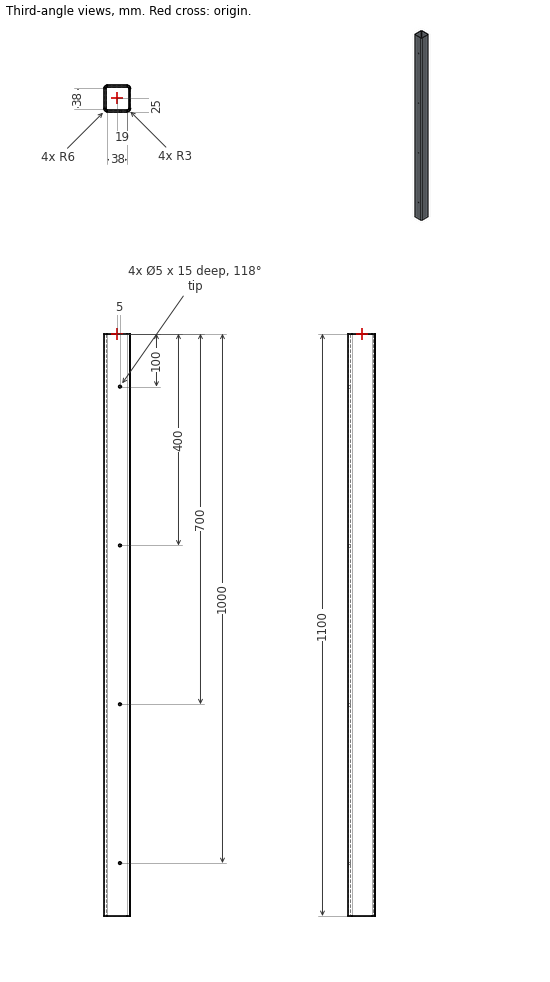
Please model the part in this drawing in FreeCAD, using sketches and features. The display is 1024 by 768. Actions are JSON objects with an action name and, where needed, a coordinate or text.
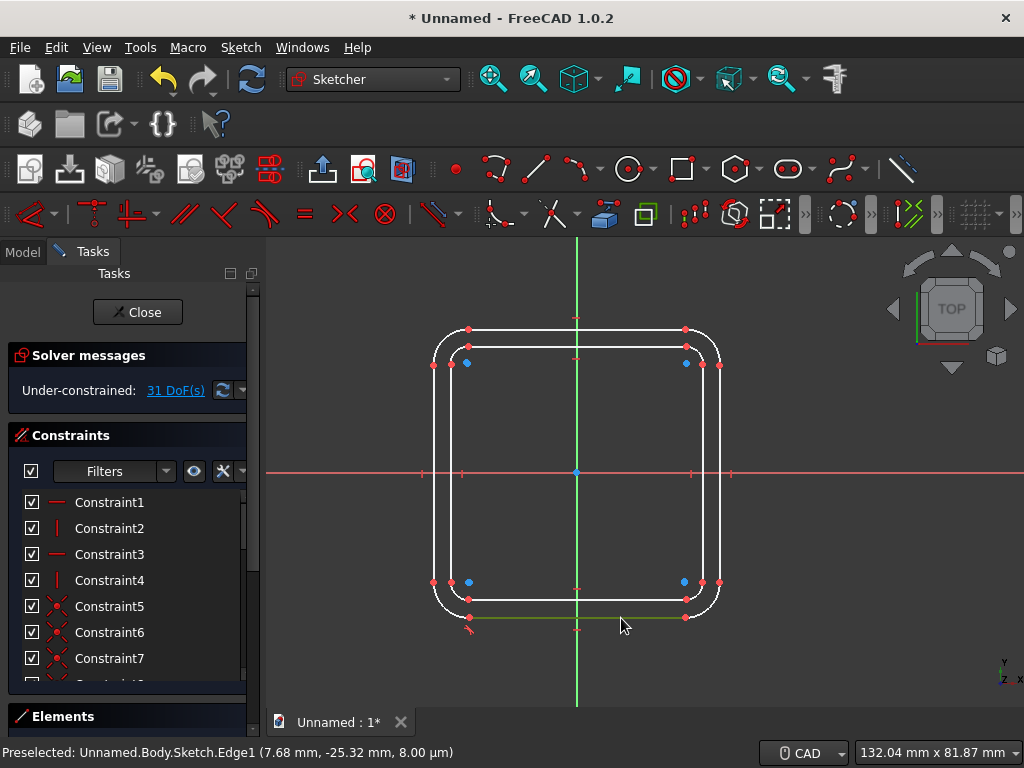
{"action": "left_click", "coordinate": [701, 614]}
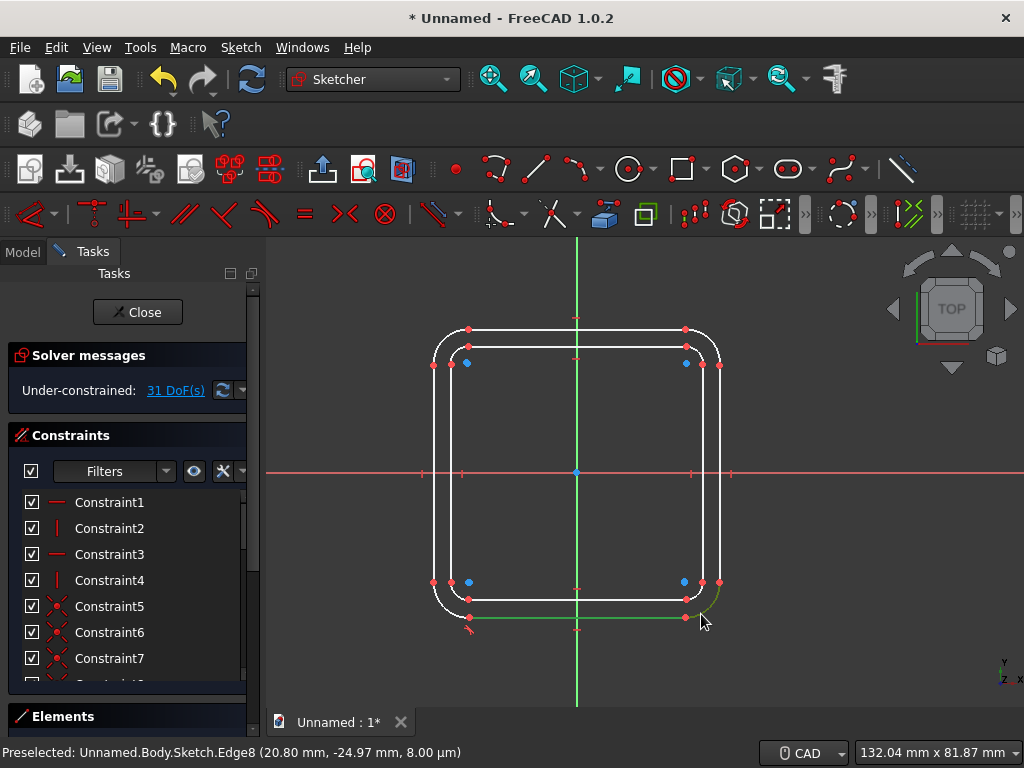
{"action": "left_click", "coordinate": [266, 214]}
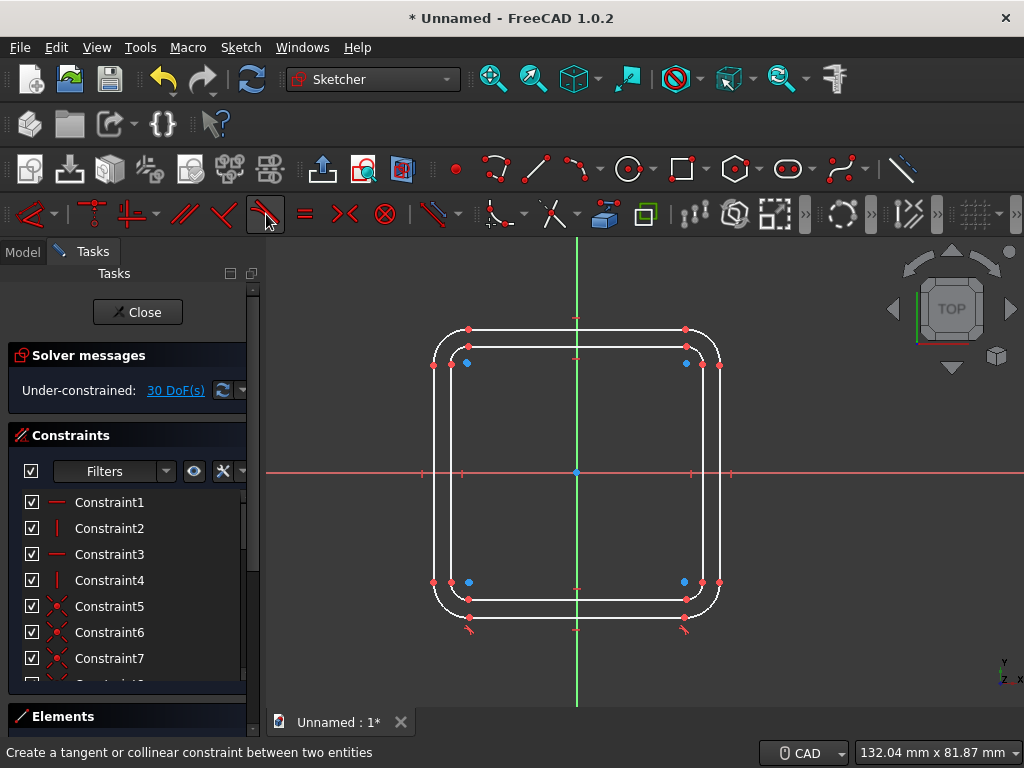
{"action": "left_click", "coordinate": [434, 517]}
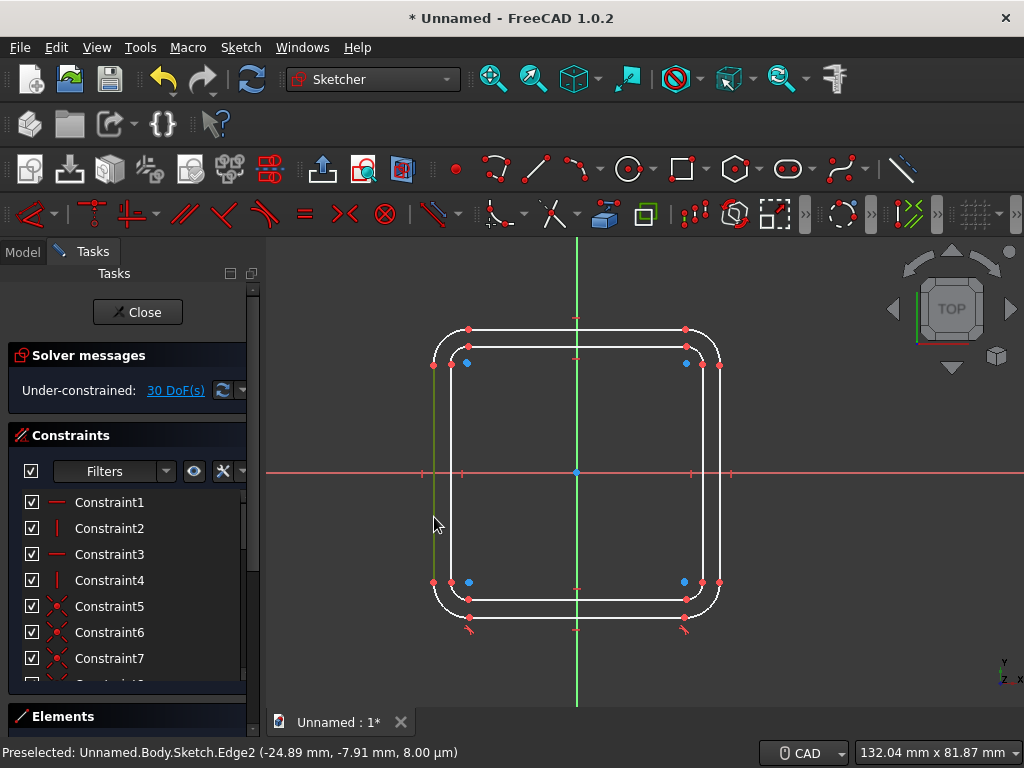
{"action": "left_click", "coordinate": [438, 599]}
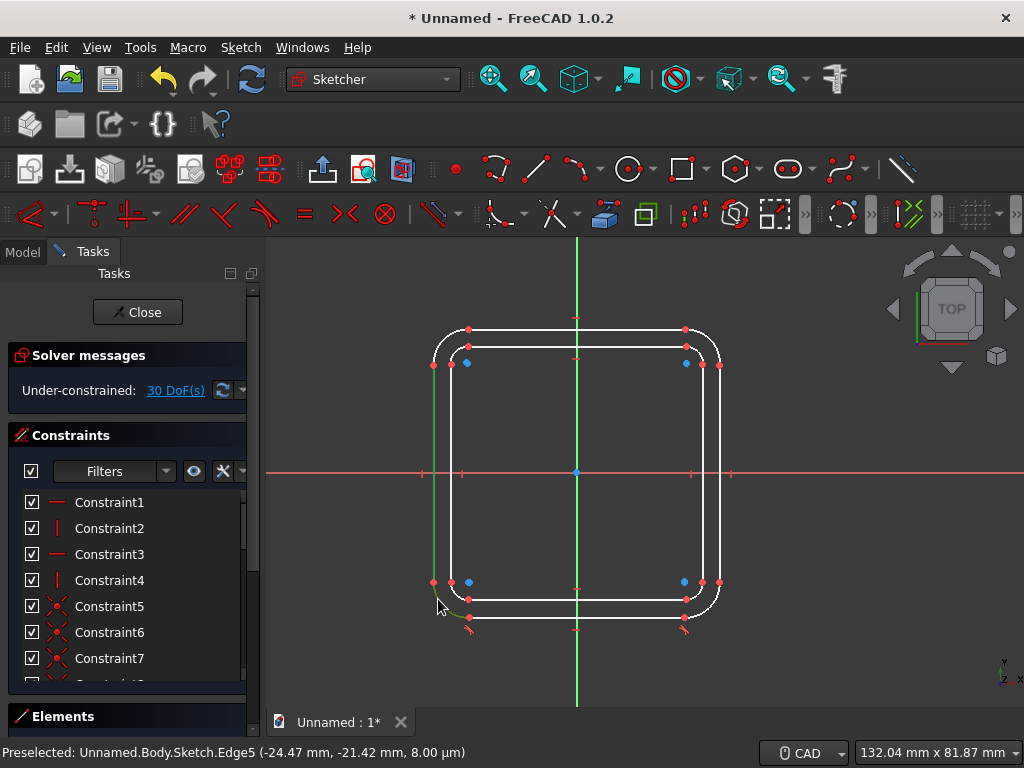
{"action": "left_click", "coordinate": [266, 214]}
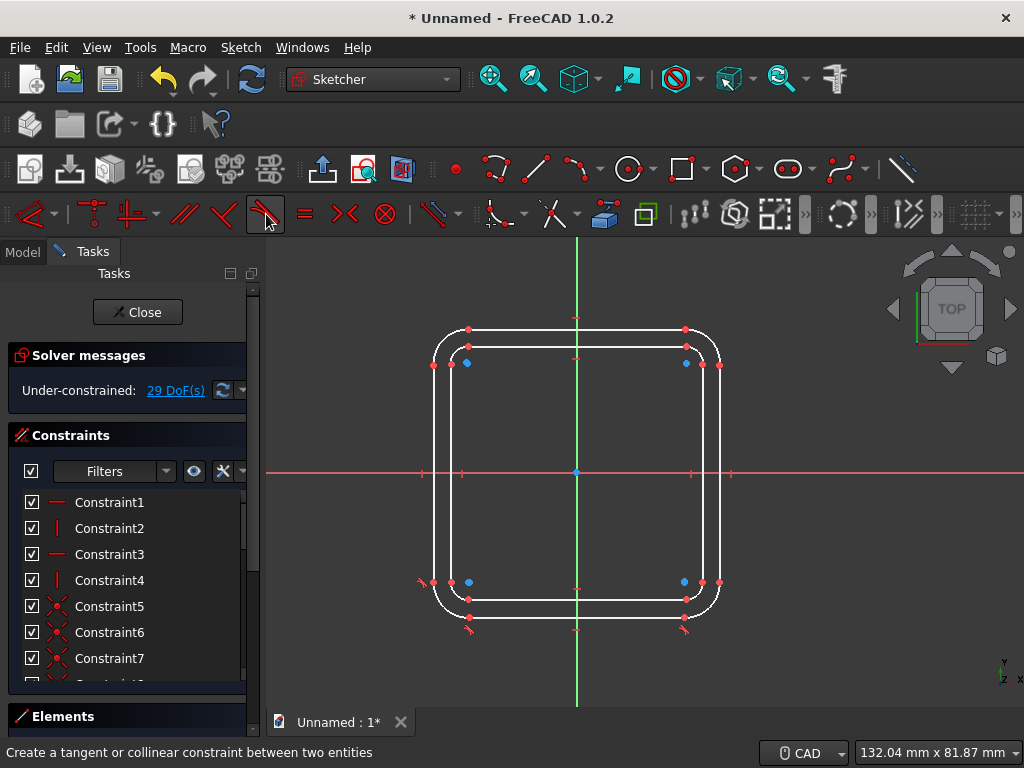
{"action": "left_click", "coordinate": [434, 517]}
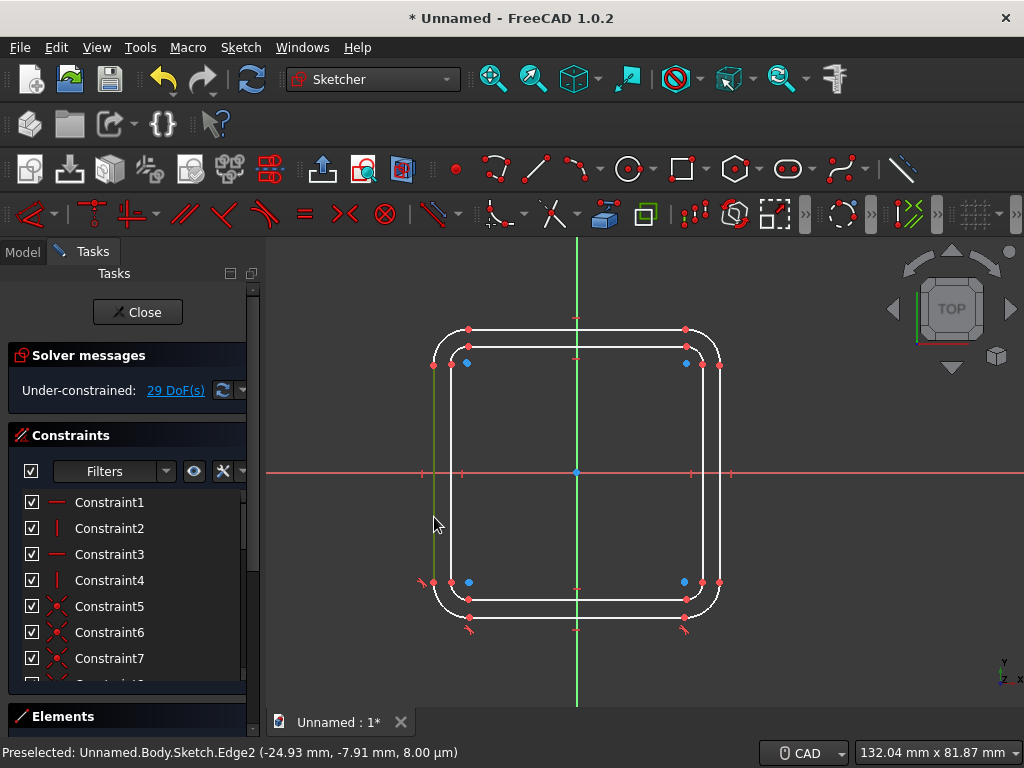
{"action": "left_click", "coordinate": [452, 333]}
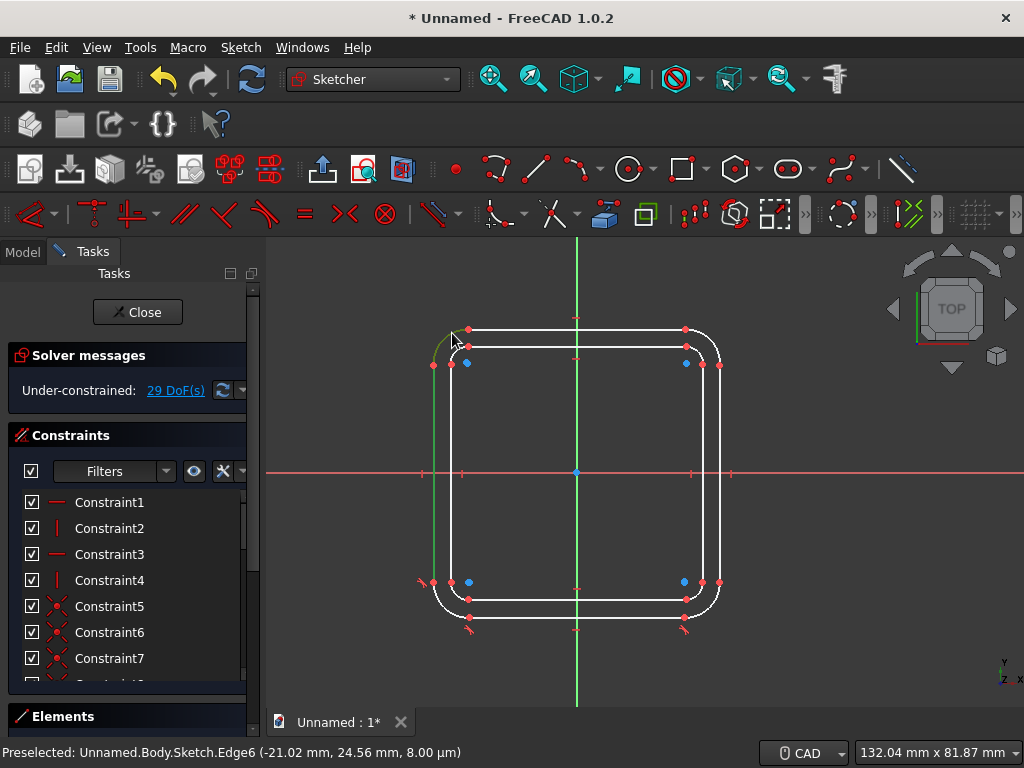
{"action": "key", "text": "t"}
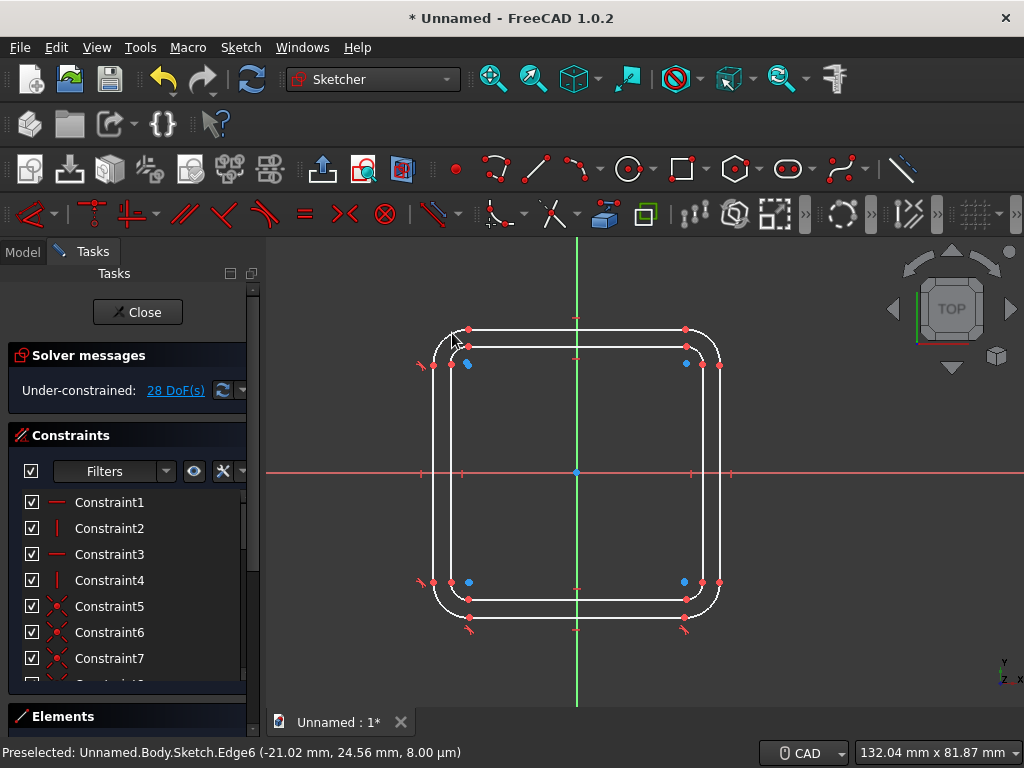
{"action": "left_click", "coordinate": [533, 330]}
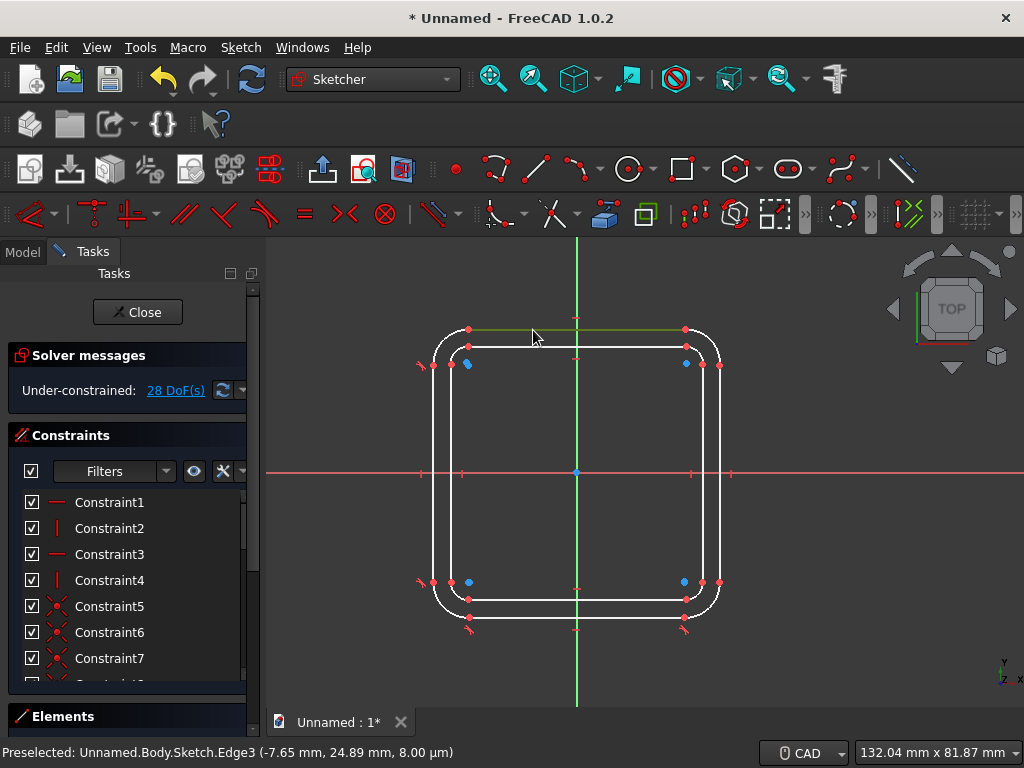
{"action": "left_click", "coordinate": [452, 334]}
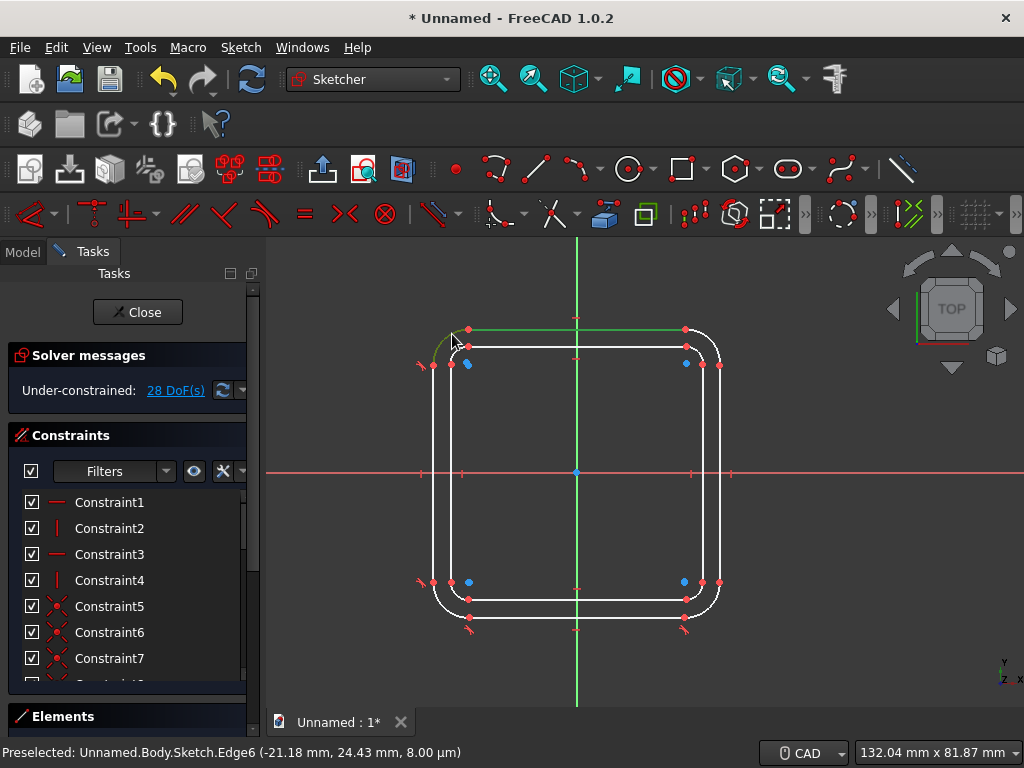
{"action": "key", "text": "t"}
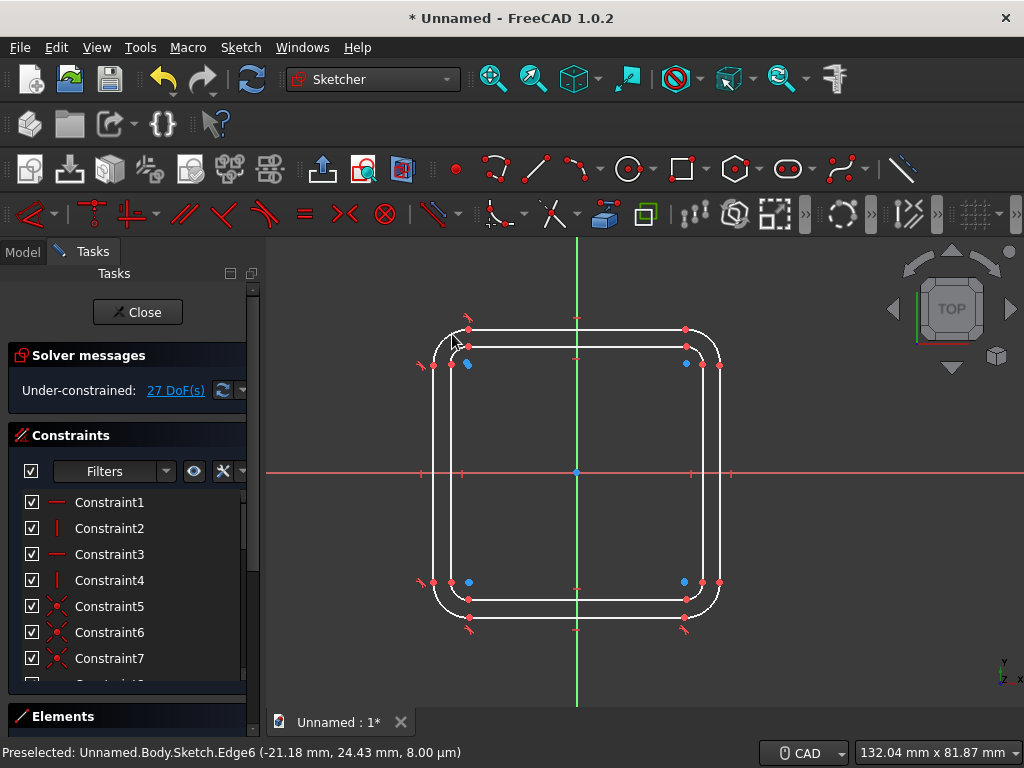
{"action": "left_click", "coordinate": [534, 330]}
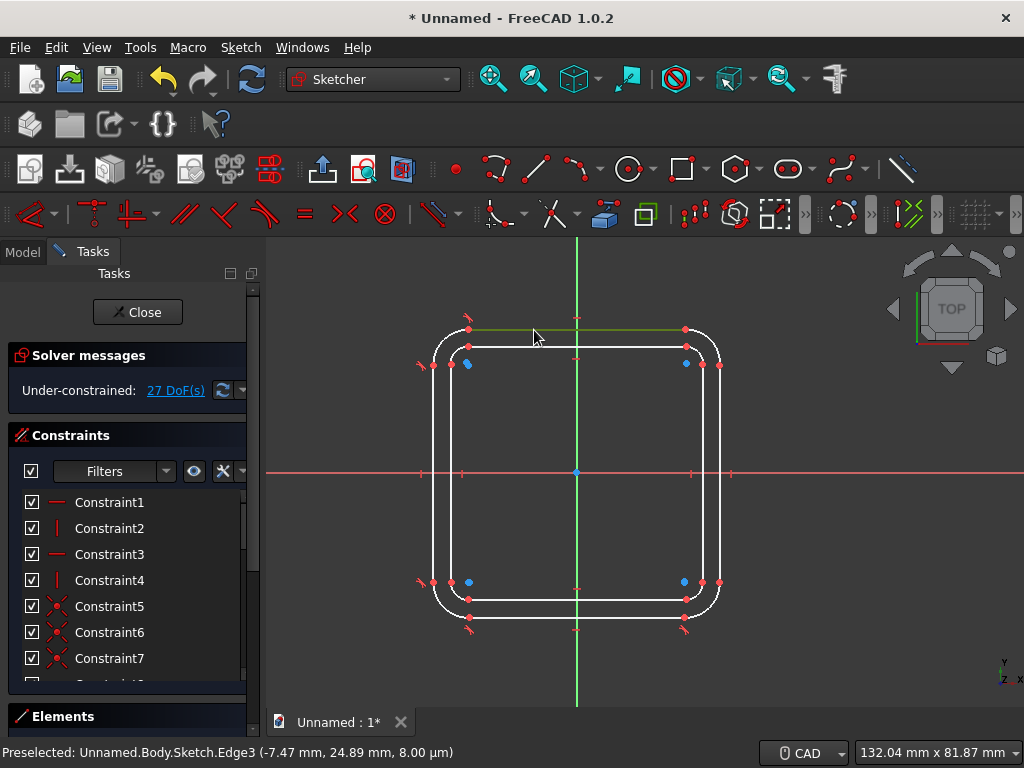
{"action": "left_click", "coordinate": [717, 349]}